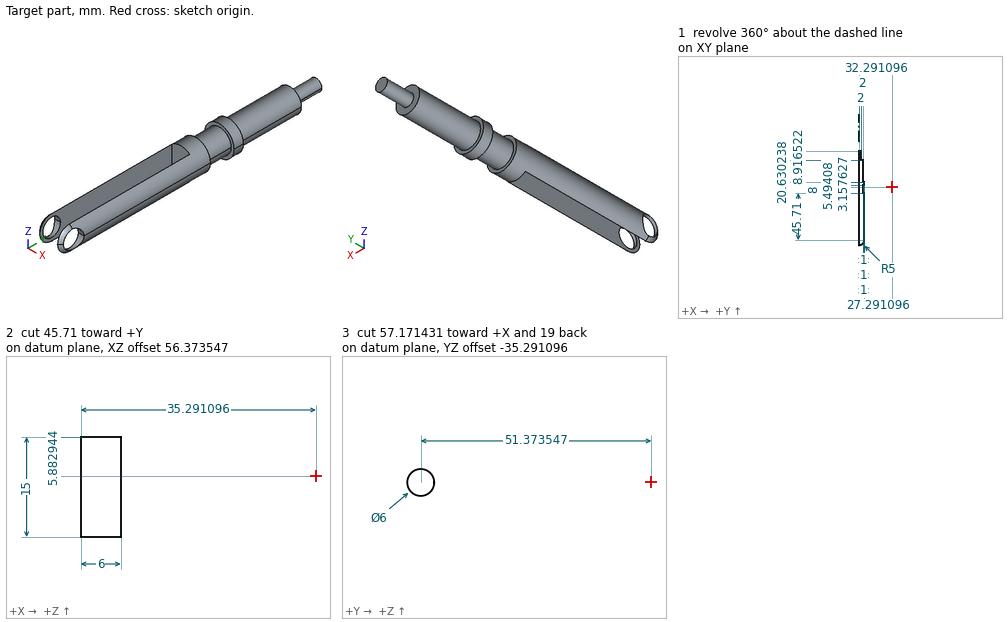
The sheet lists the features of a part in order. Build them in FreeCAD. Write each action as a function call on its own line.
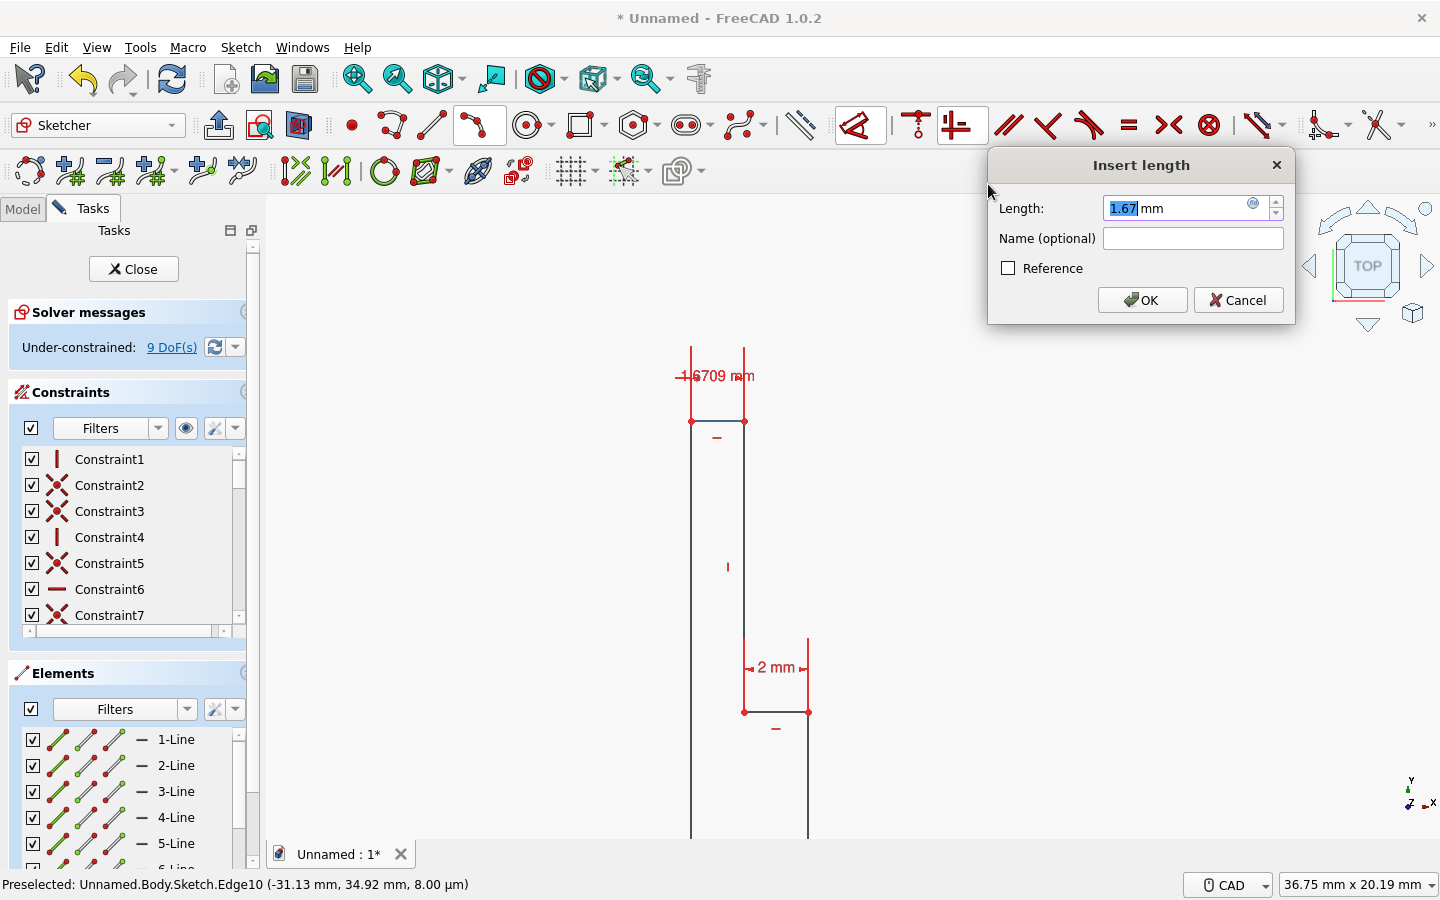
text(2)
key(Return)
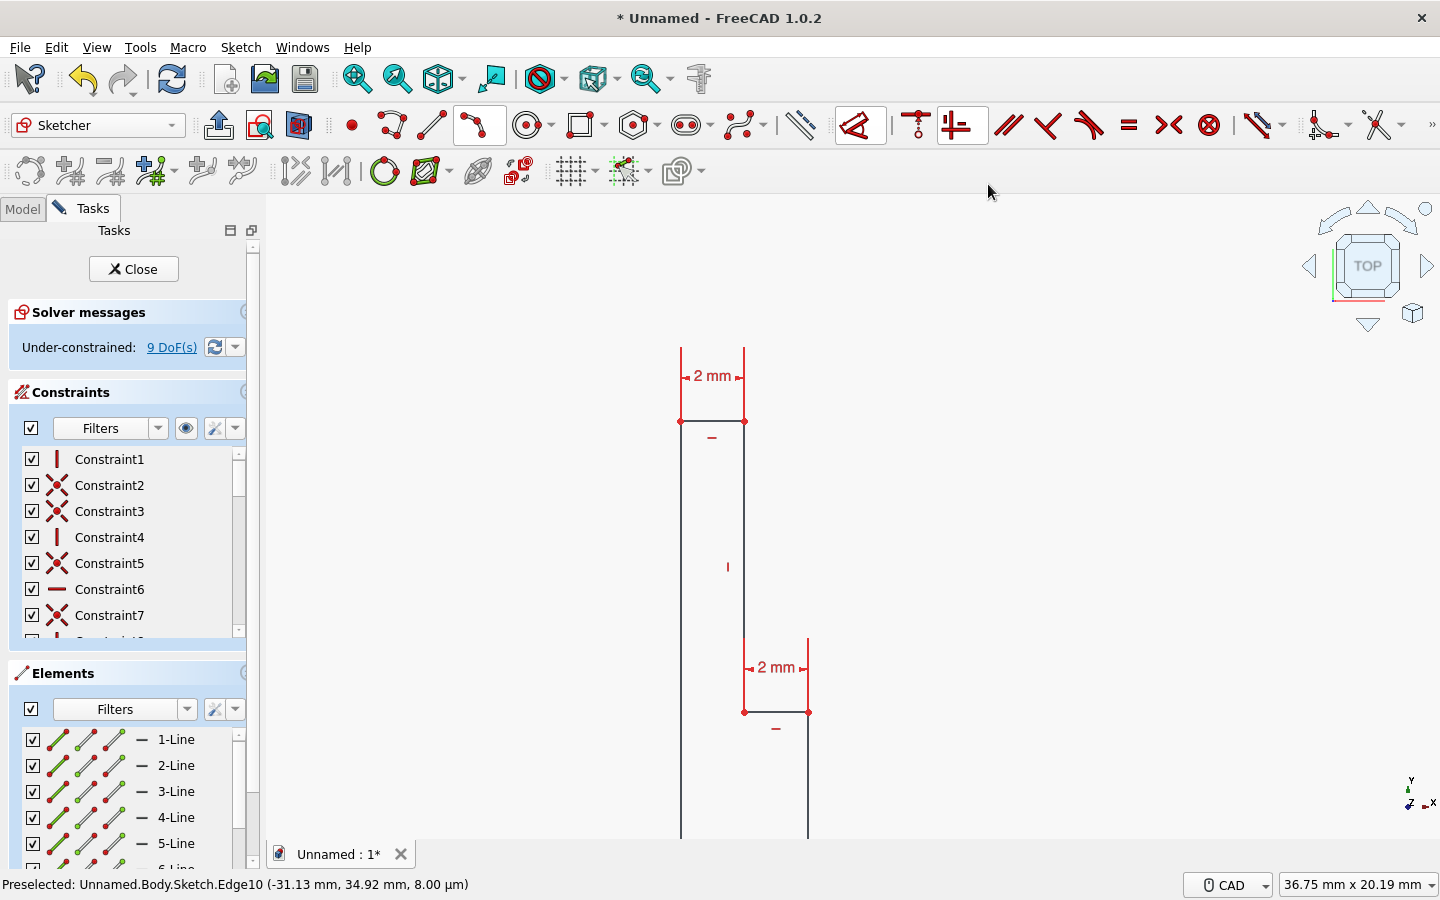
scroll(732, 420, down, 11)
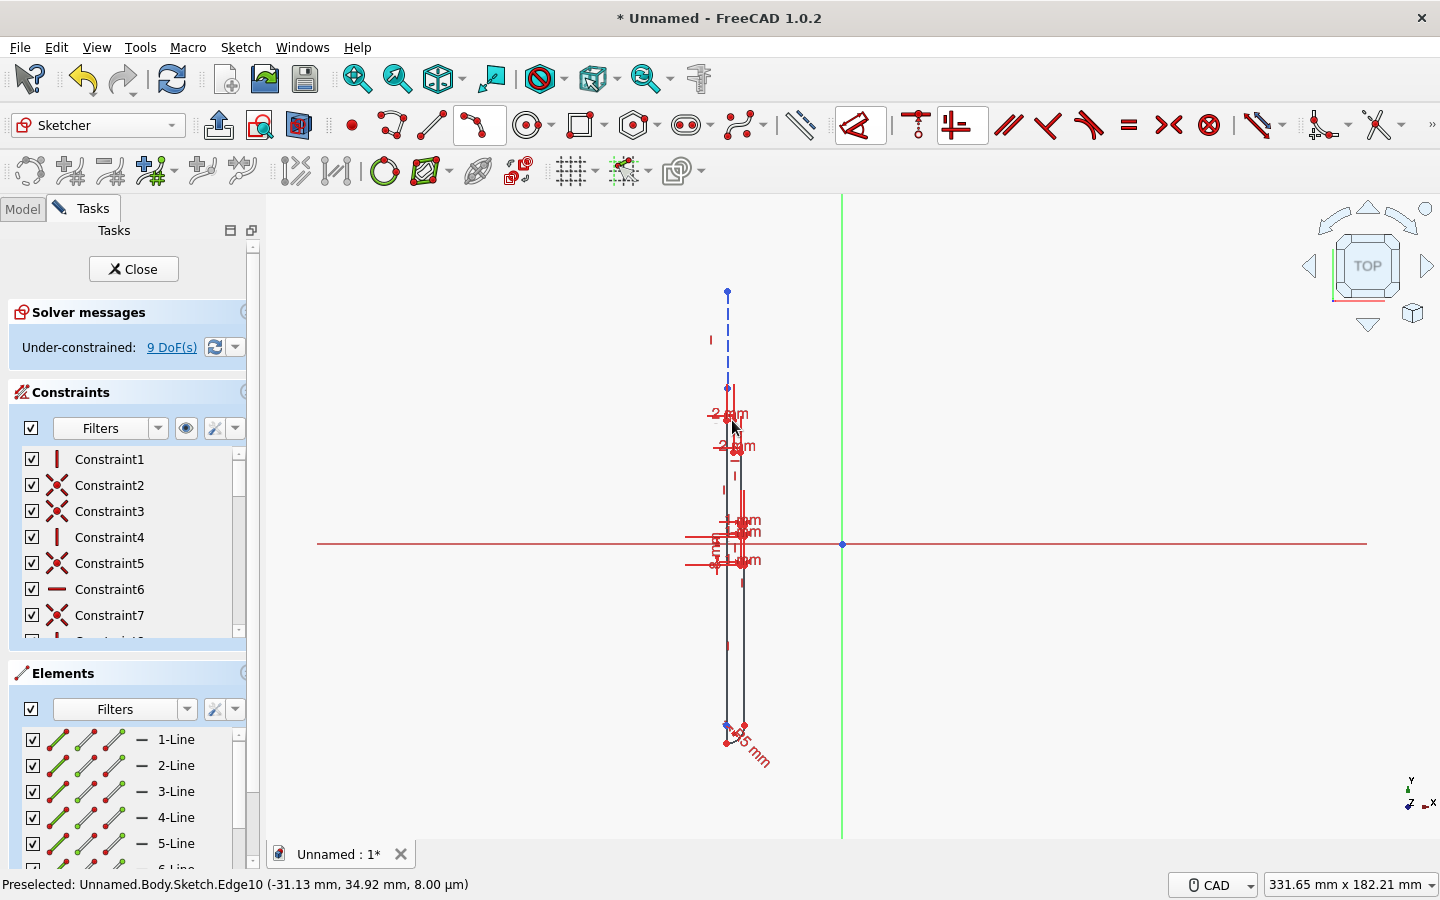
click(744, 678)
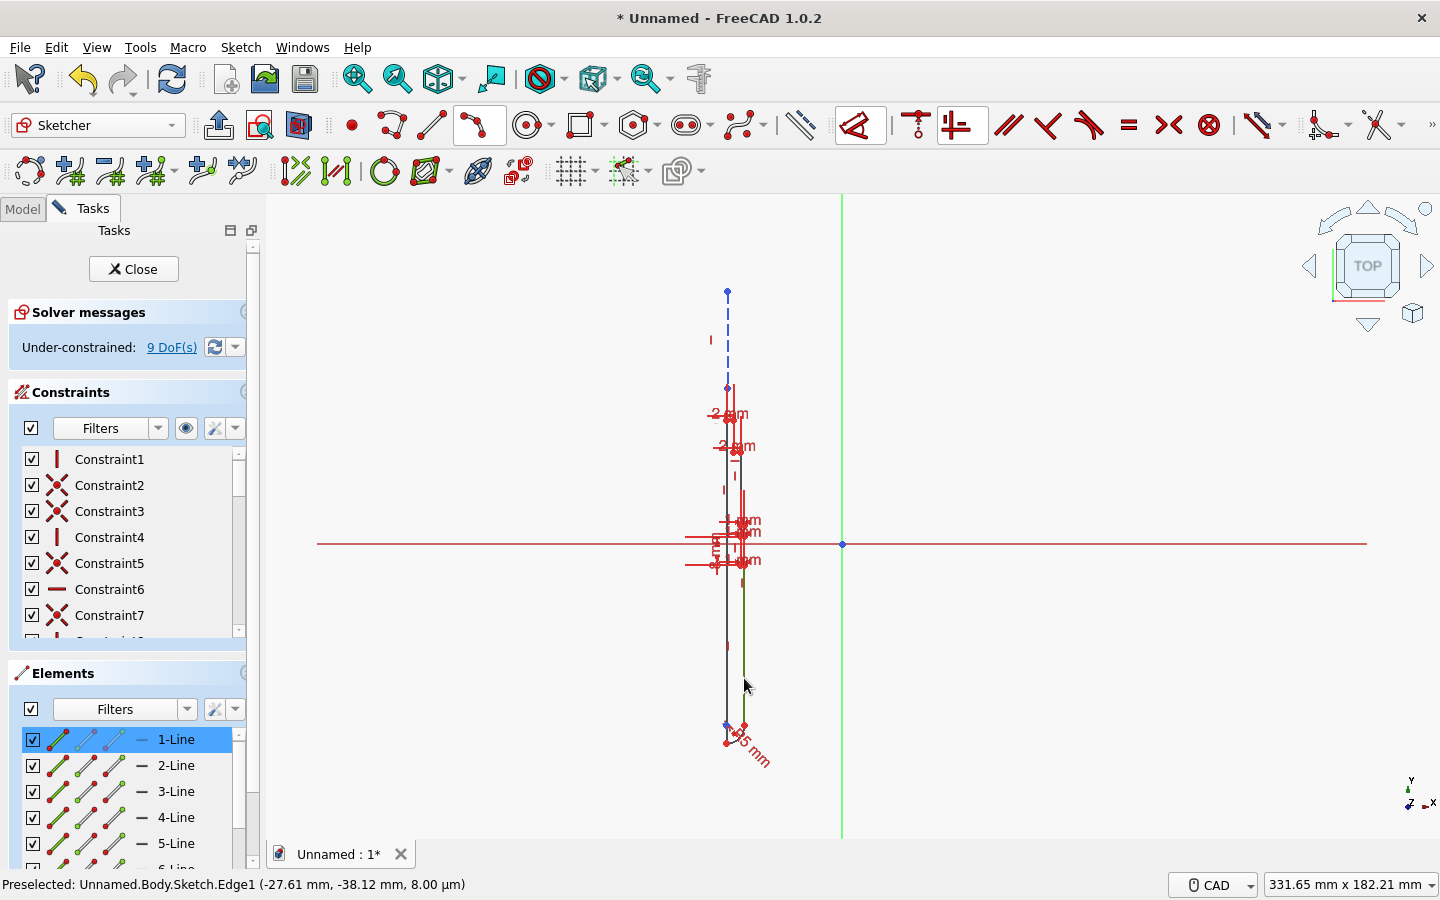
key(i)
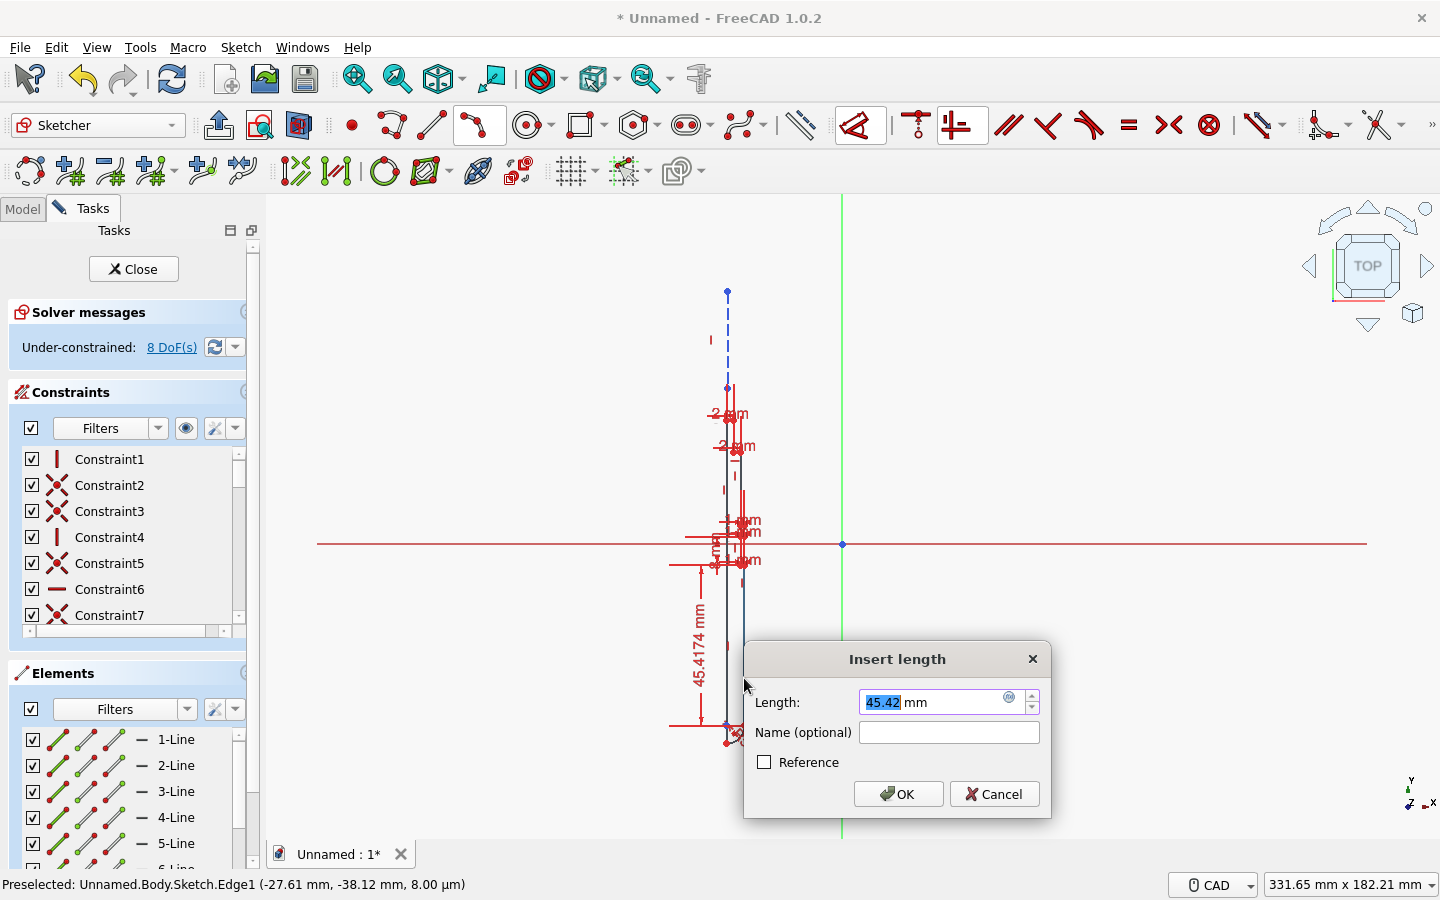
text(45.71)
key(Return)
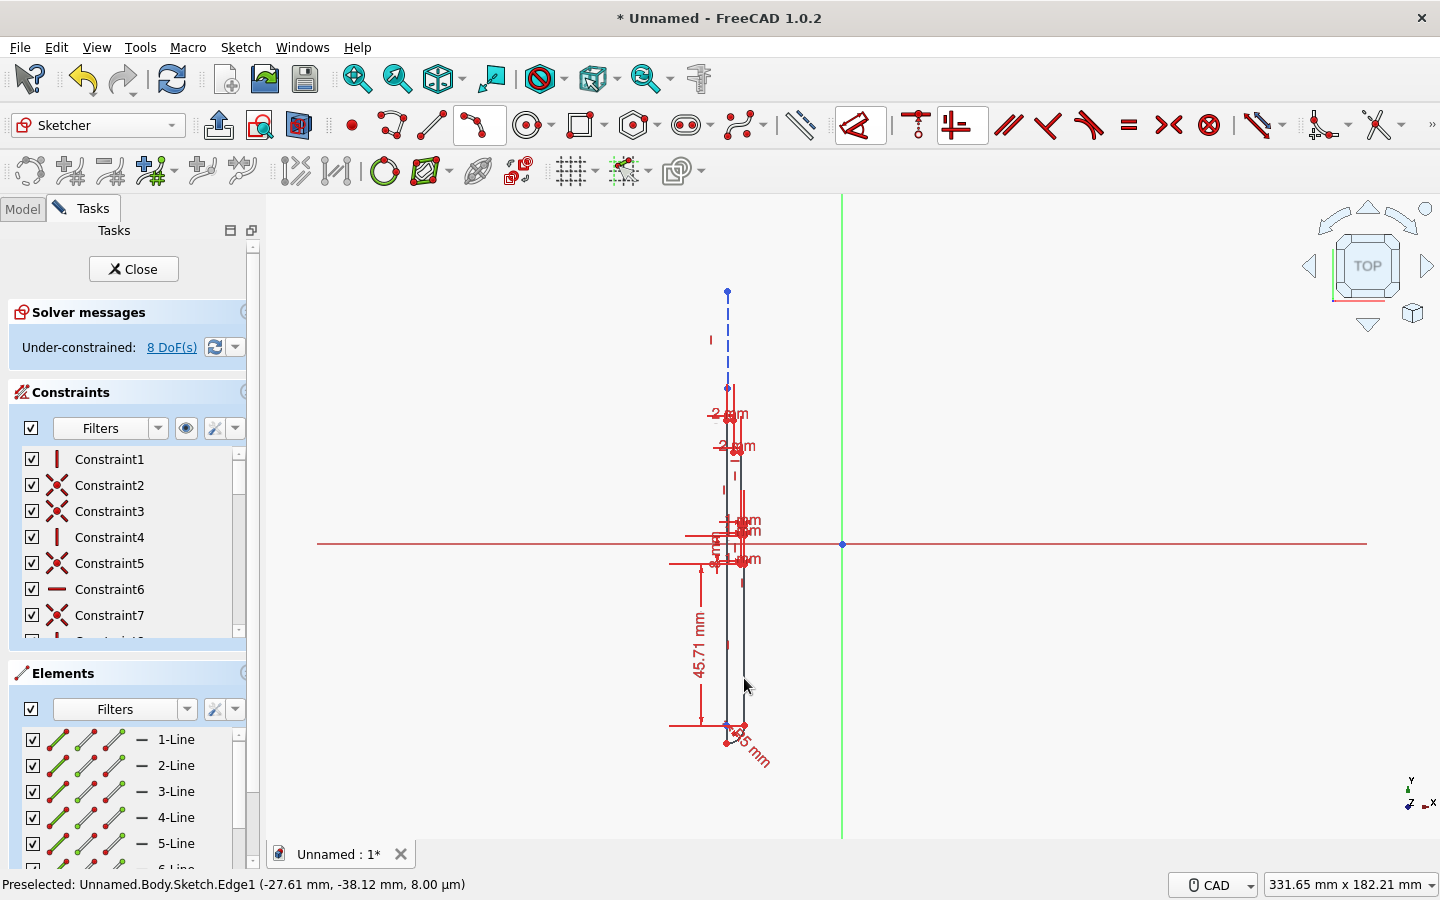
scroll(744, 531, up, 7)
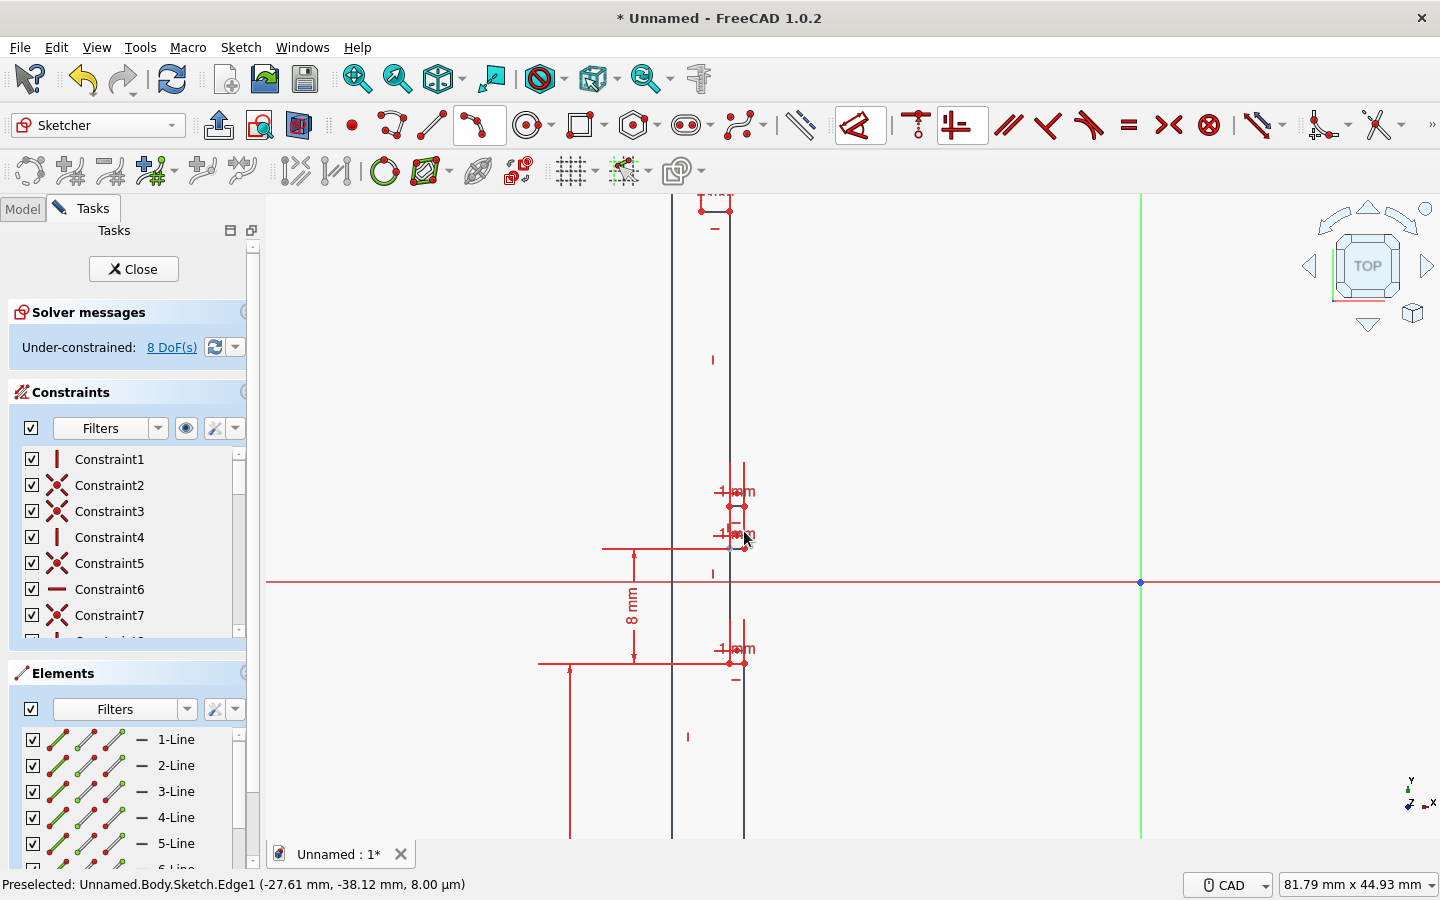
click(744, 523)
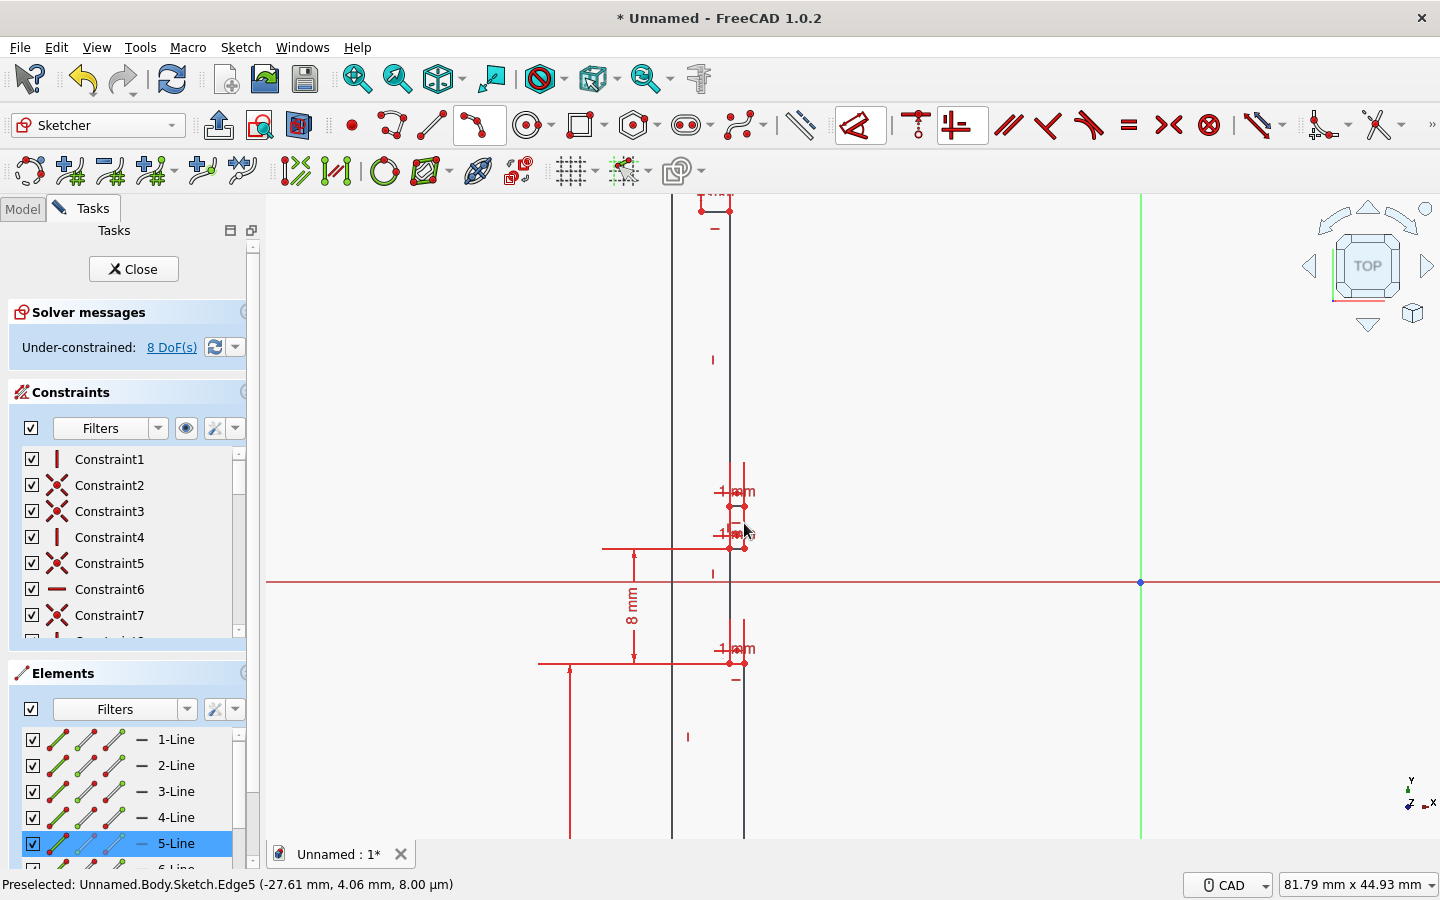
key(i)